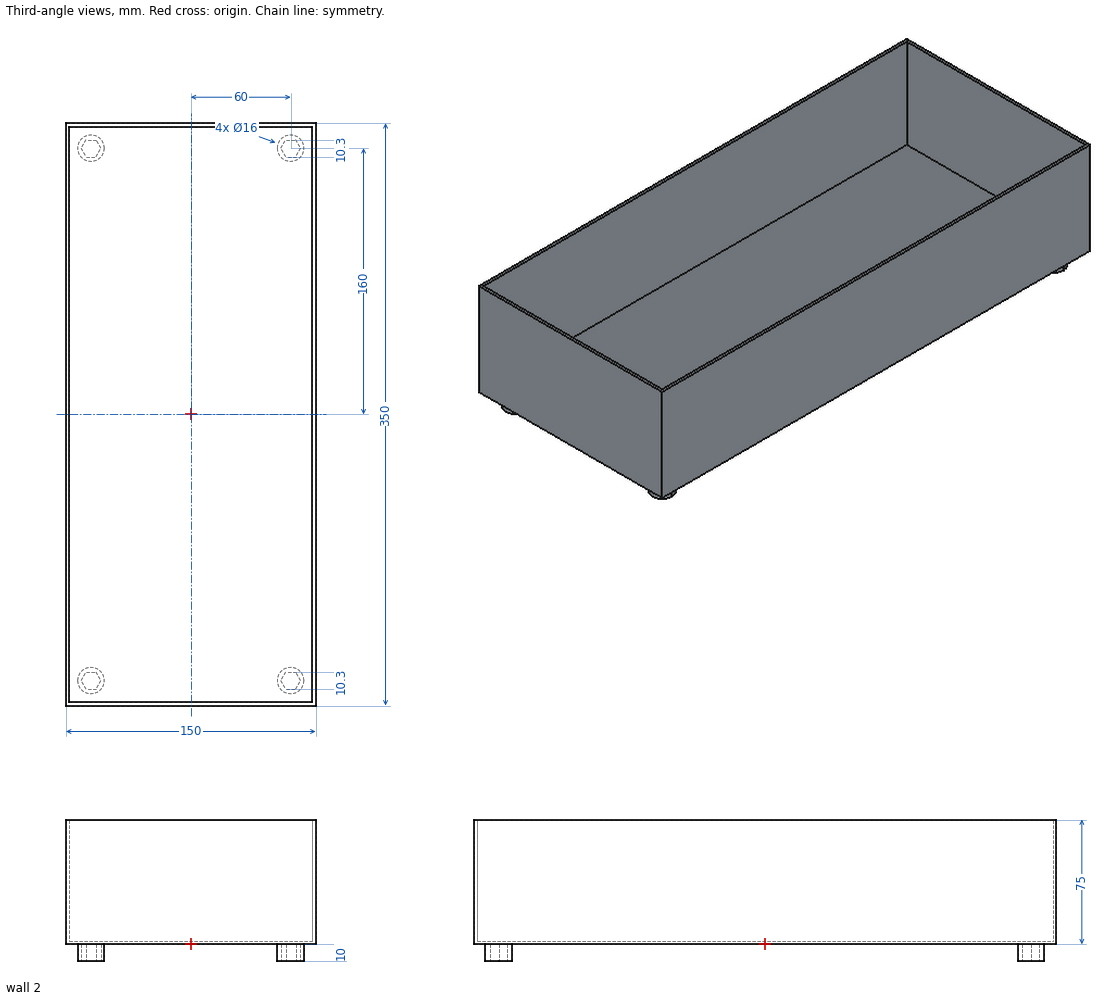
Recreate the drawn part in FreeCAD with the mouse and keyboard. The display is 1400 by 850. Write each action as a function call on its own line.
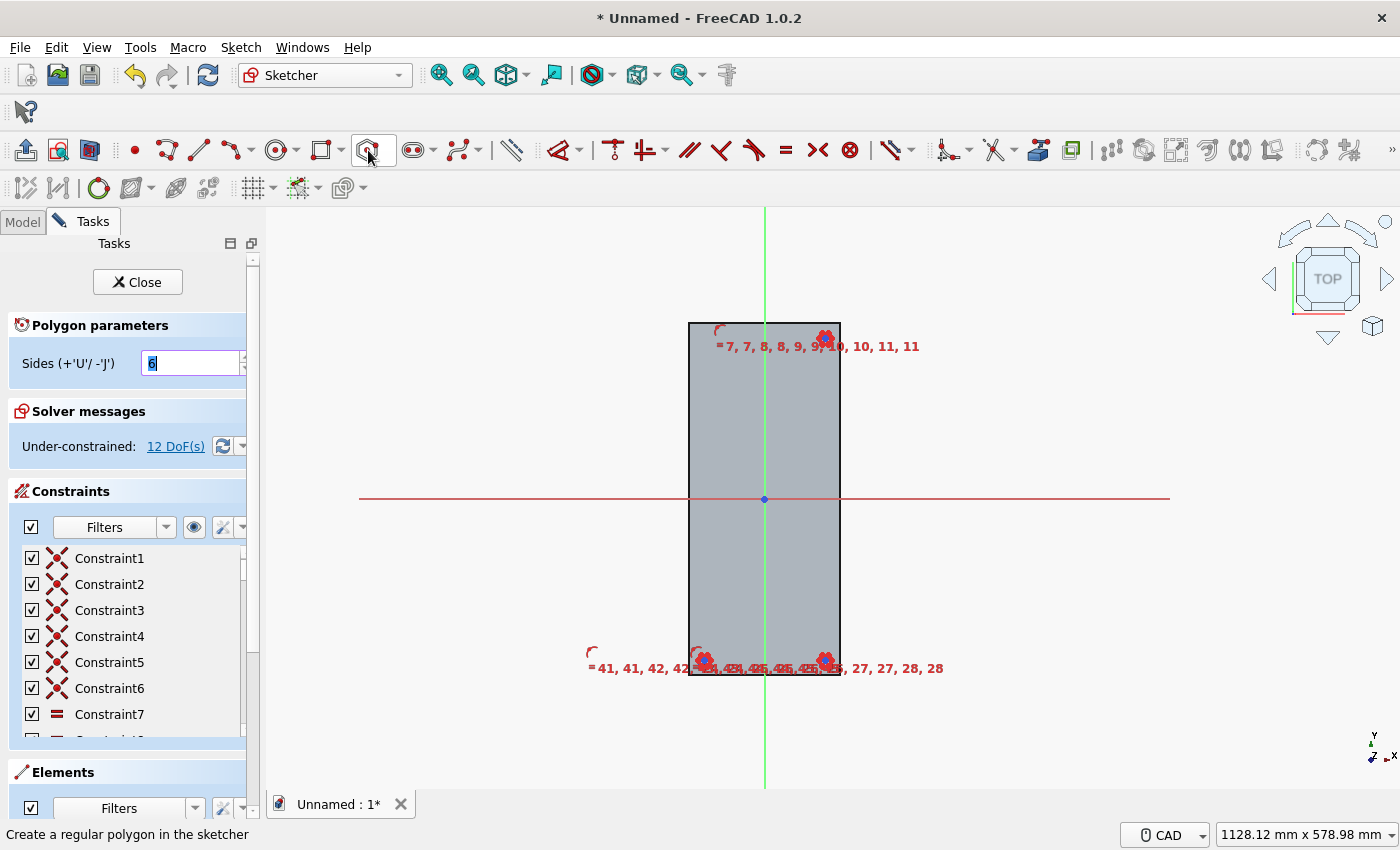
scroll(704, 338, up, 9)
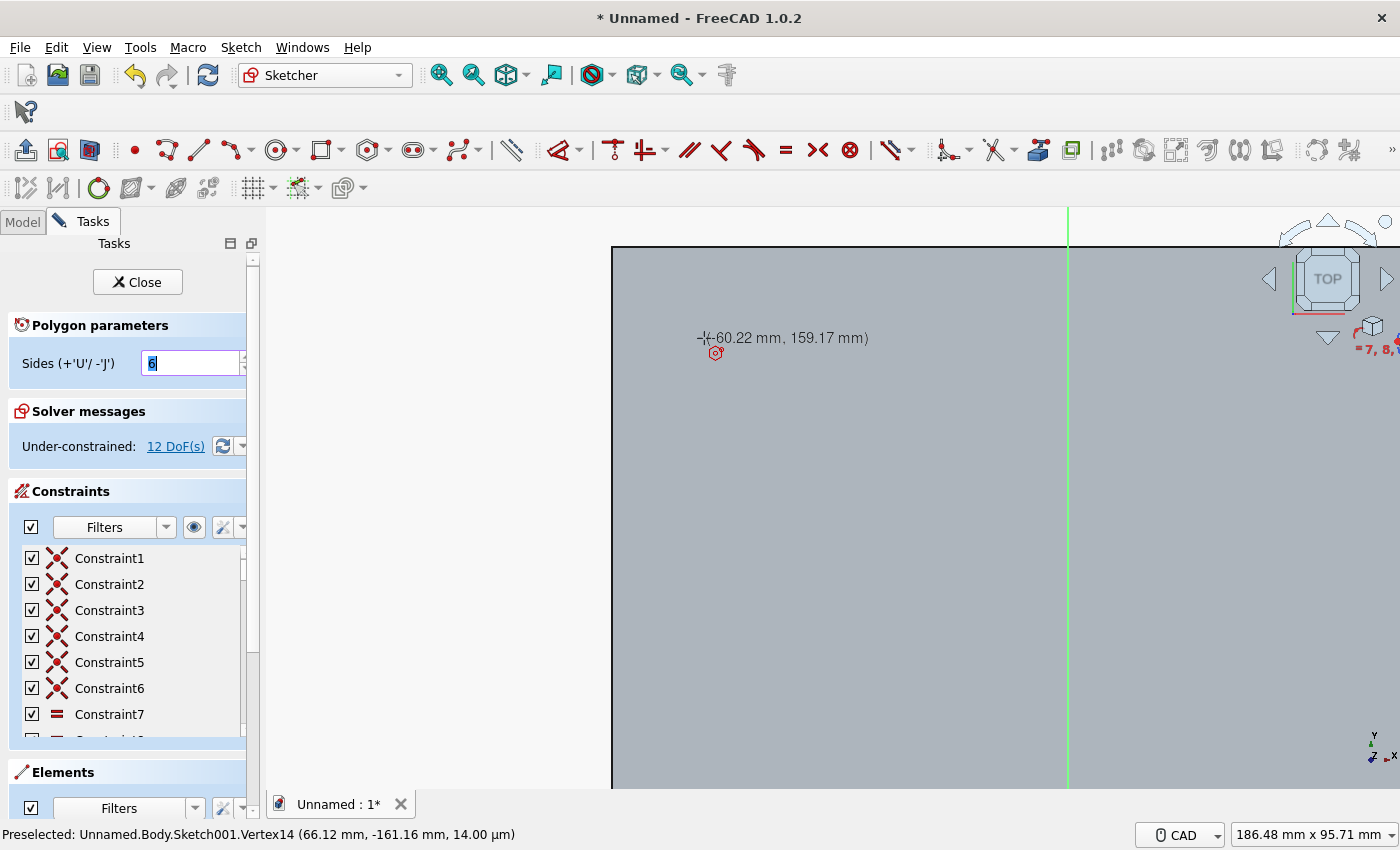
scroll(704, 337, down, 9)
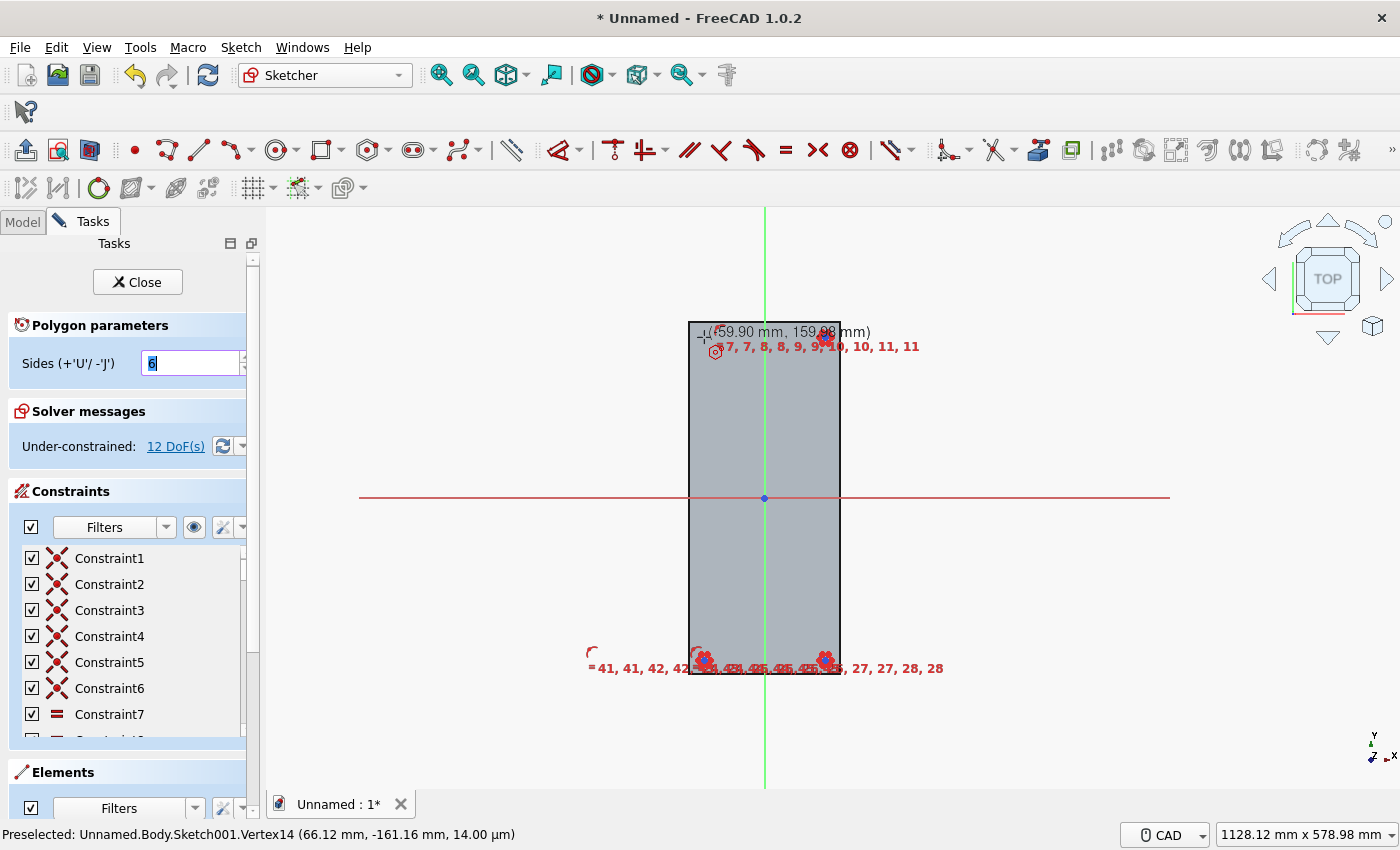
click(704, 337)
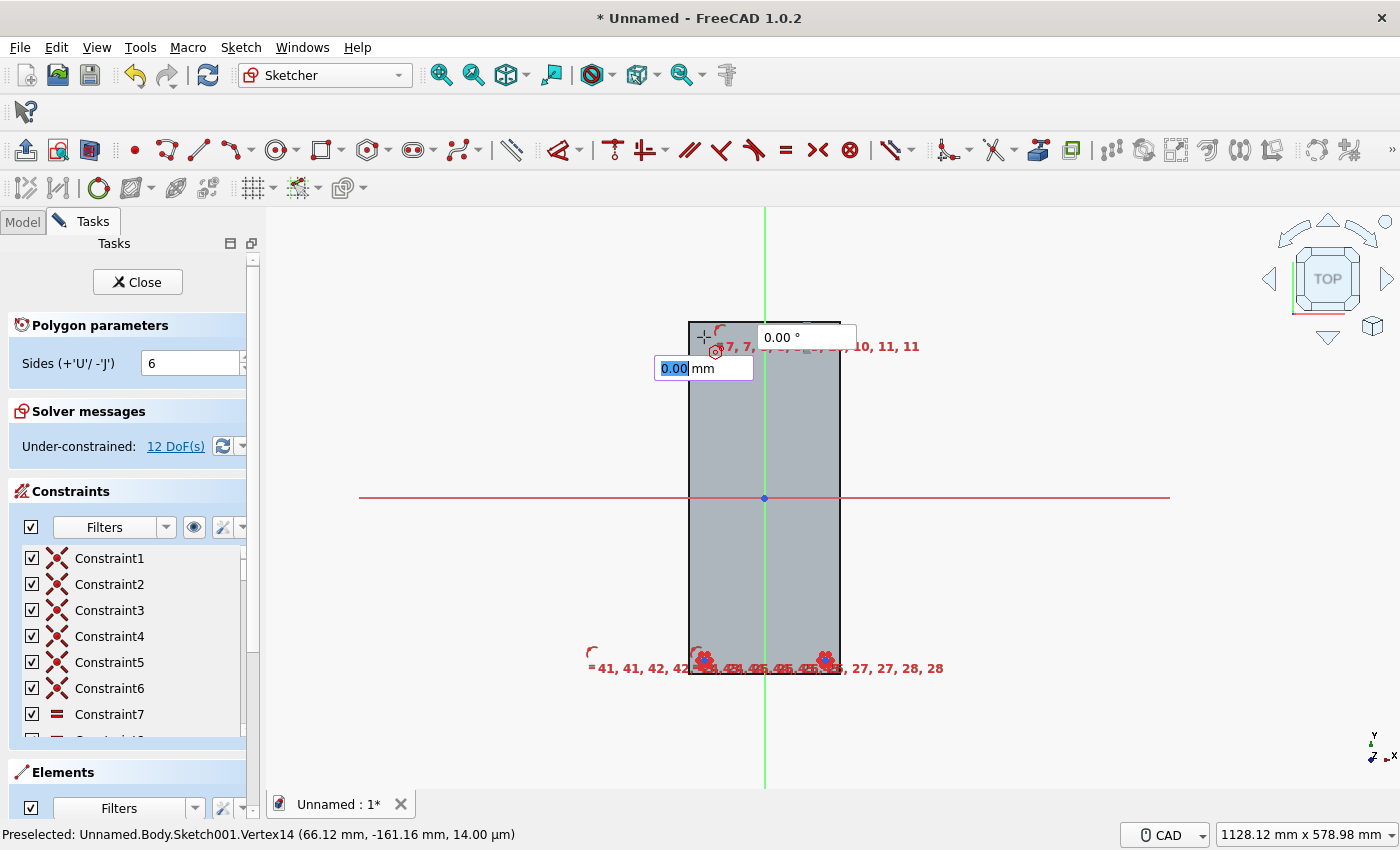
click(698, 337)
key(Escape)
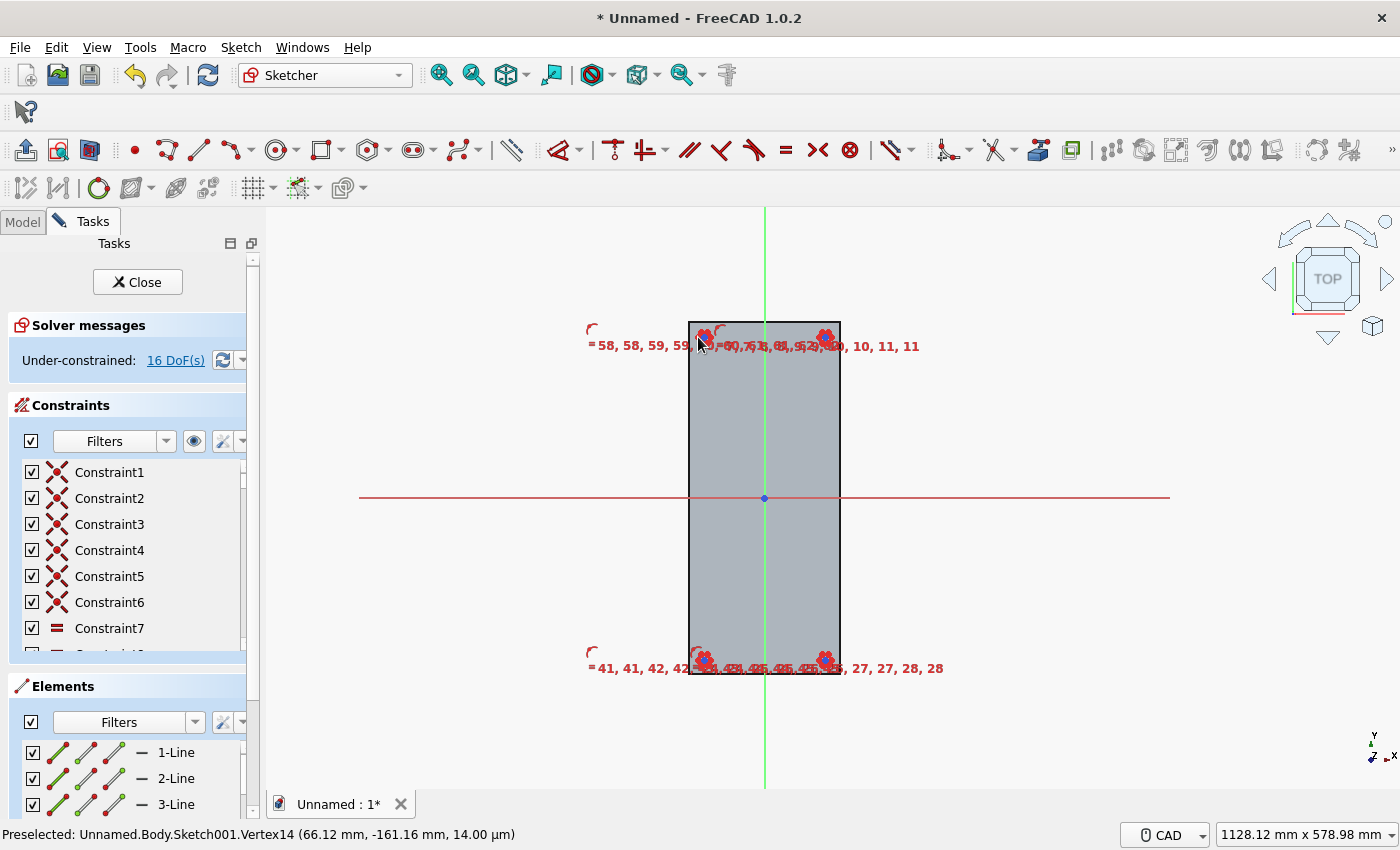
click(276, 150)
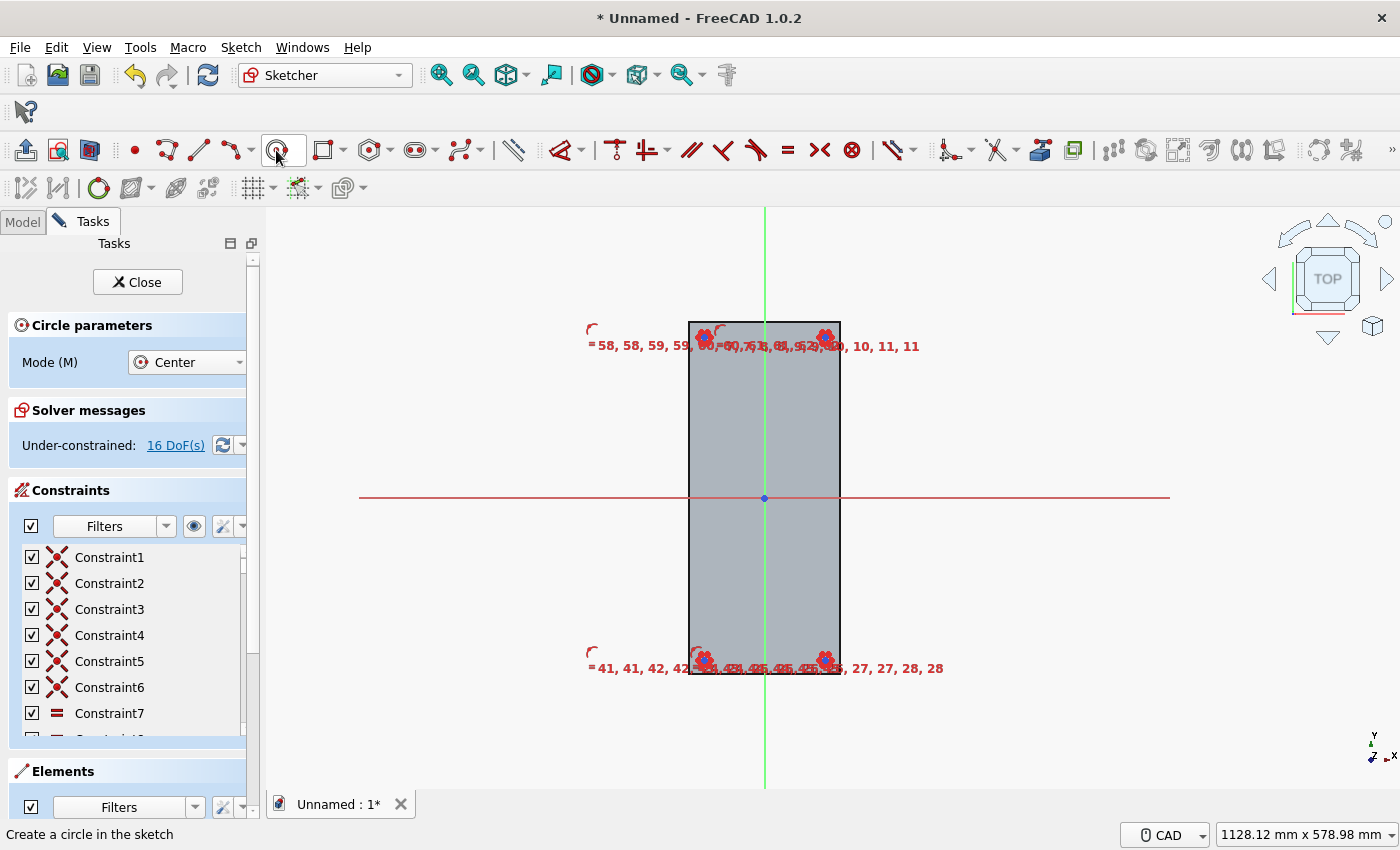
scroll(825, 337, up, 6)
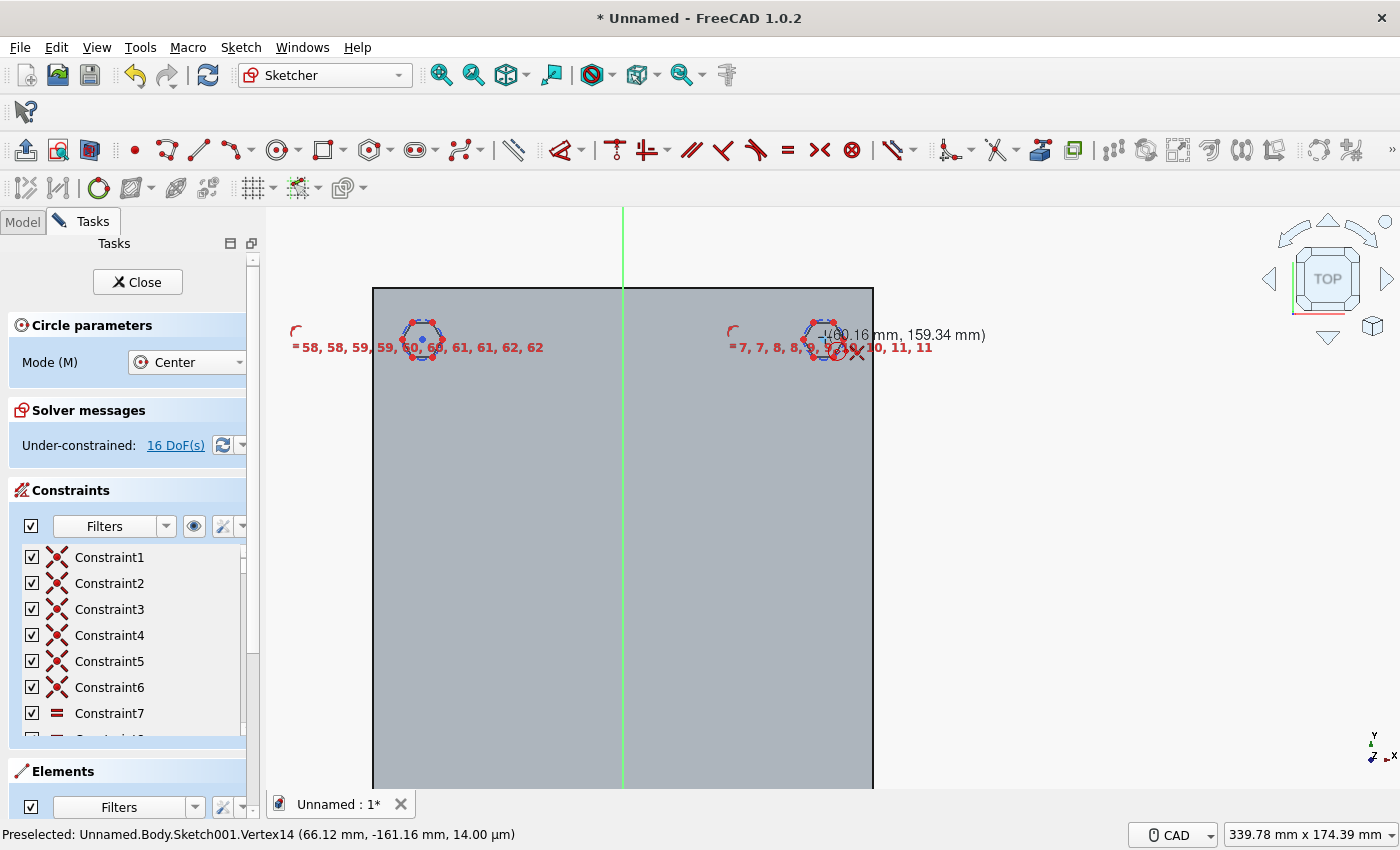
click(824, 340)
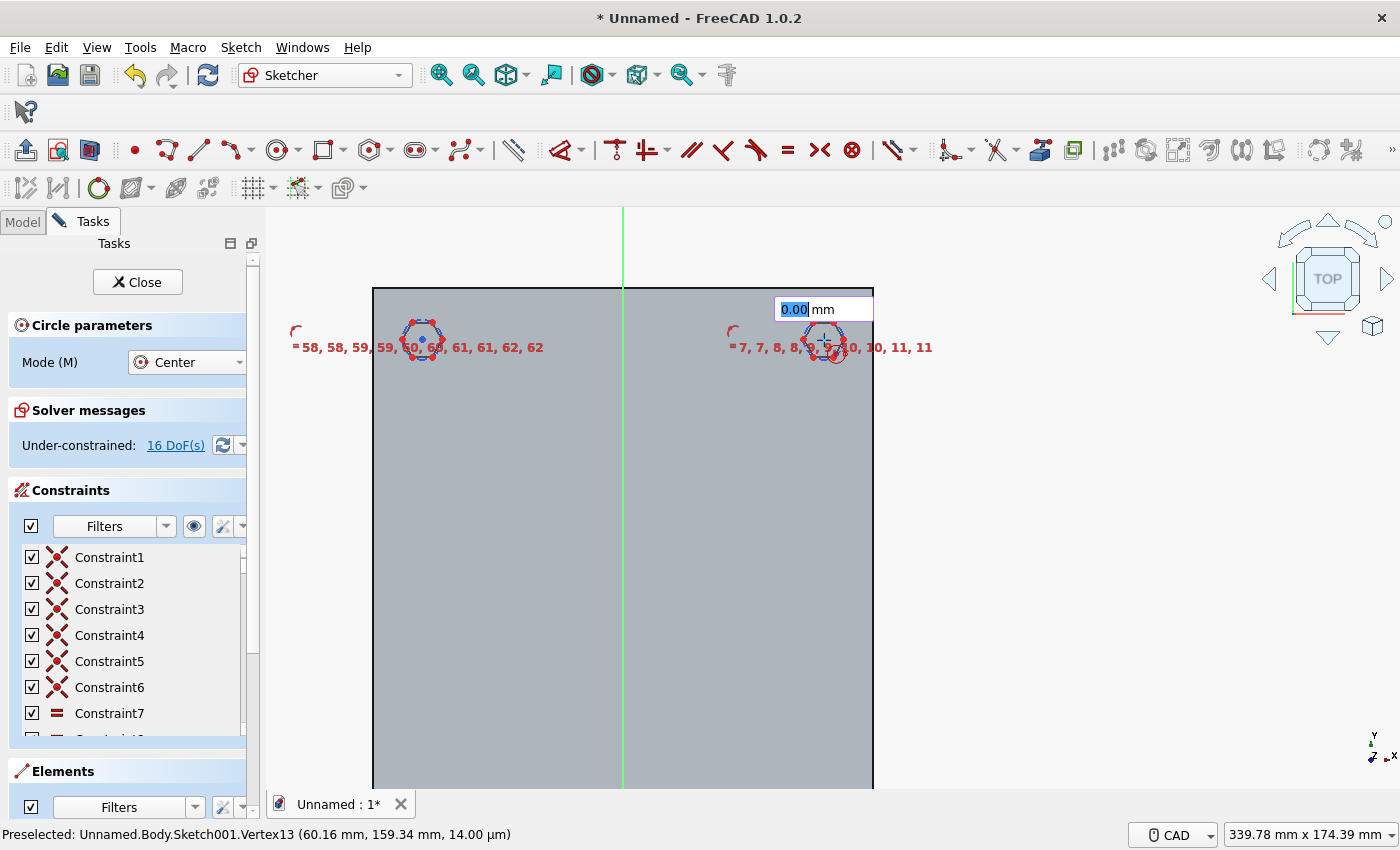
scroll(848, 328, up, 3)
move(848, 329)